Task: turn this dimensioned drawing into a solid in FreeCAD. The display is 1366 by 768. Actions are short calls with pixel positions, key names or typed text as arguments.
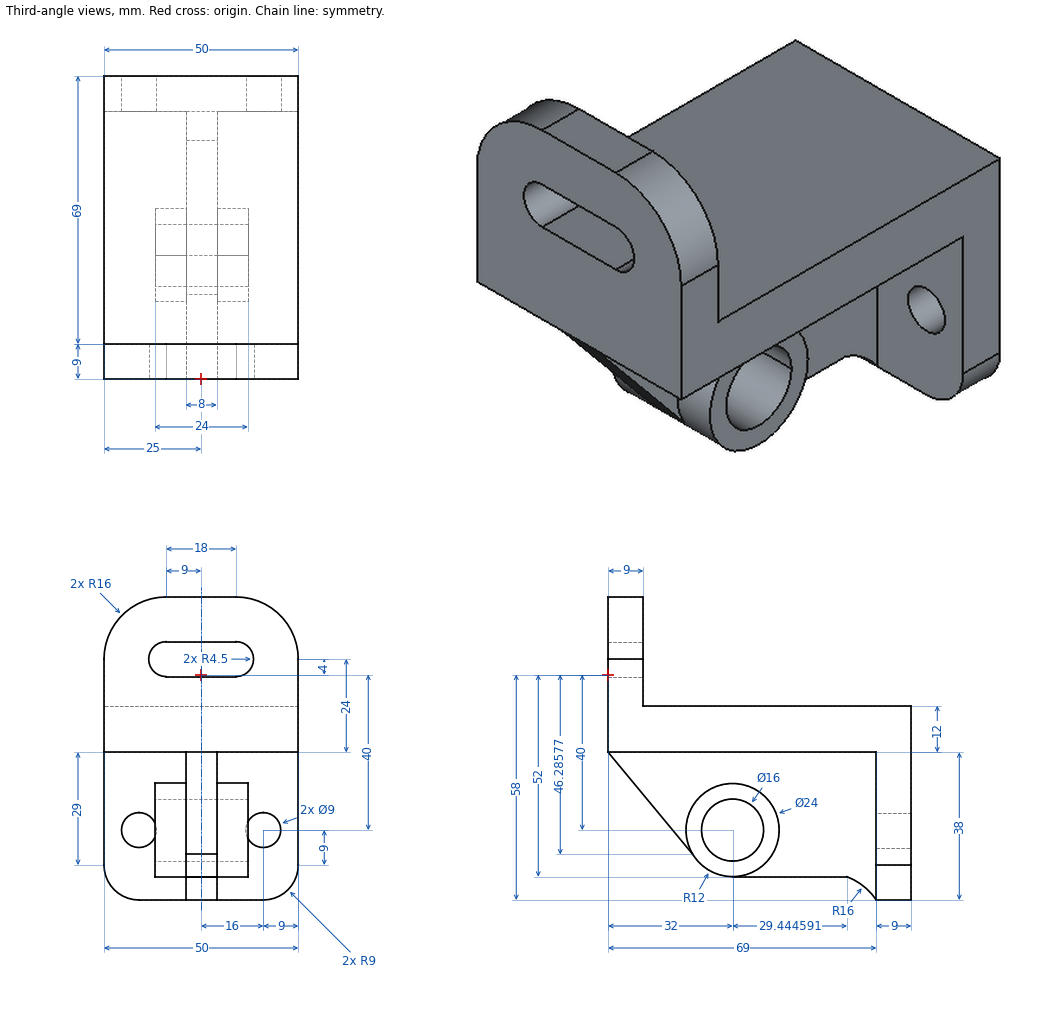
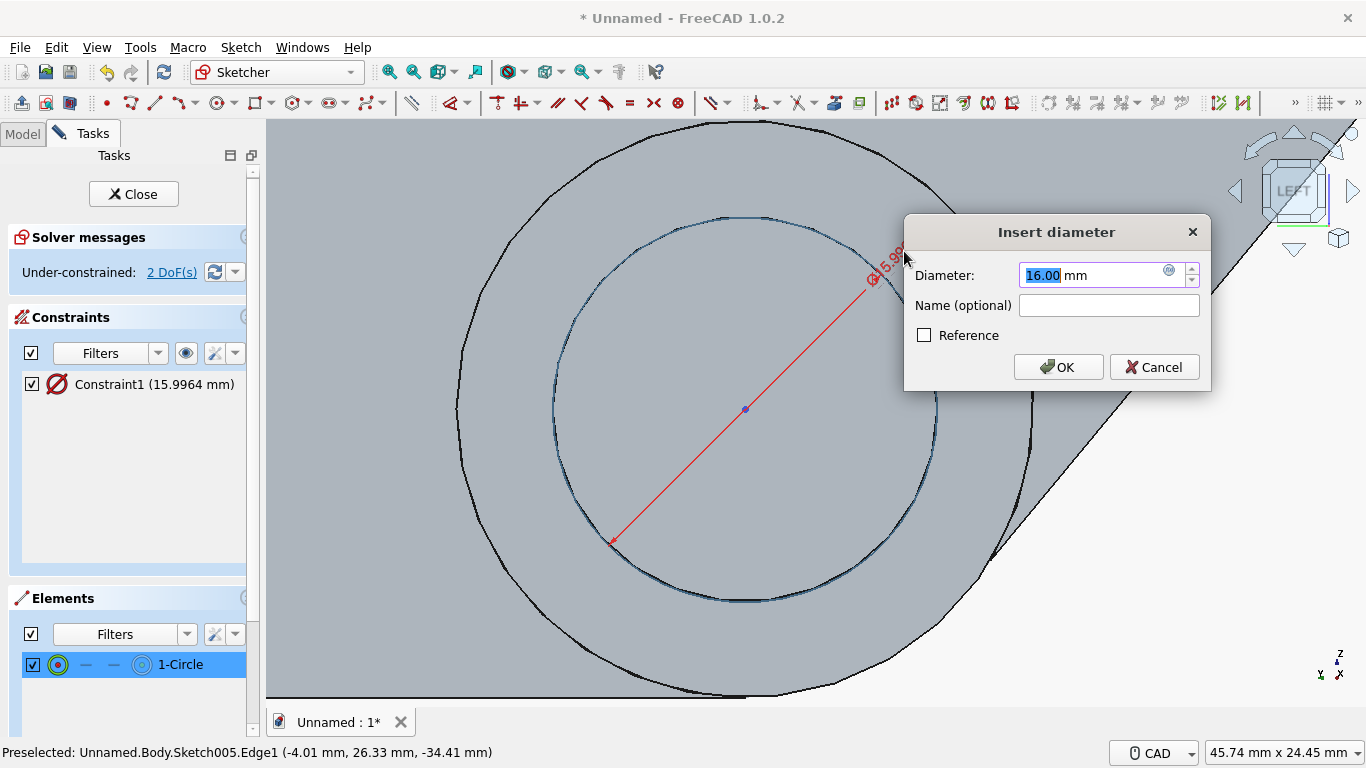
text(16)
key(Return)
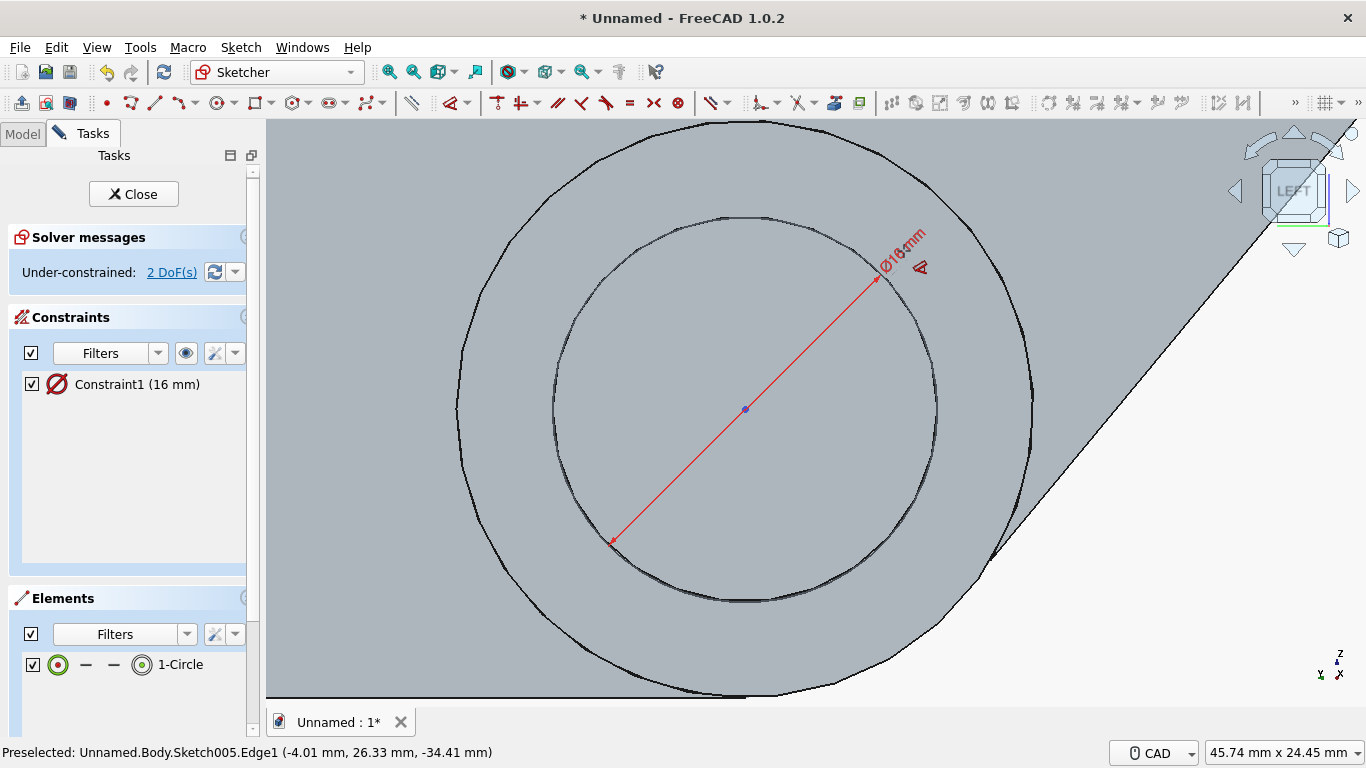
click(745, 410)
click(973, 444)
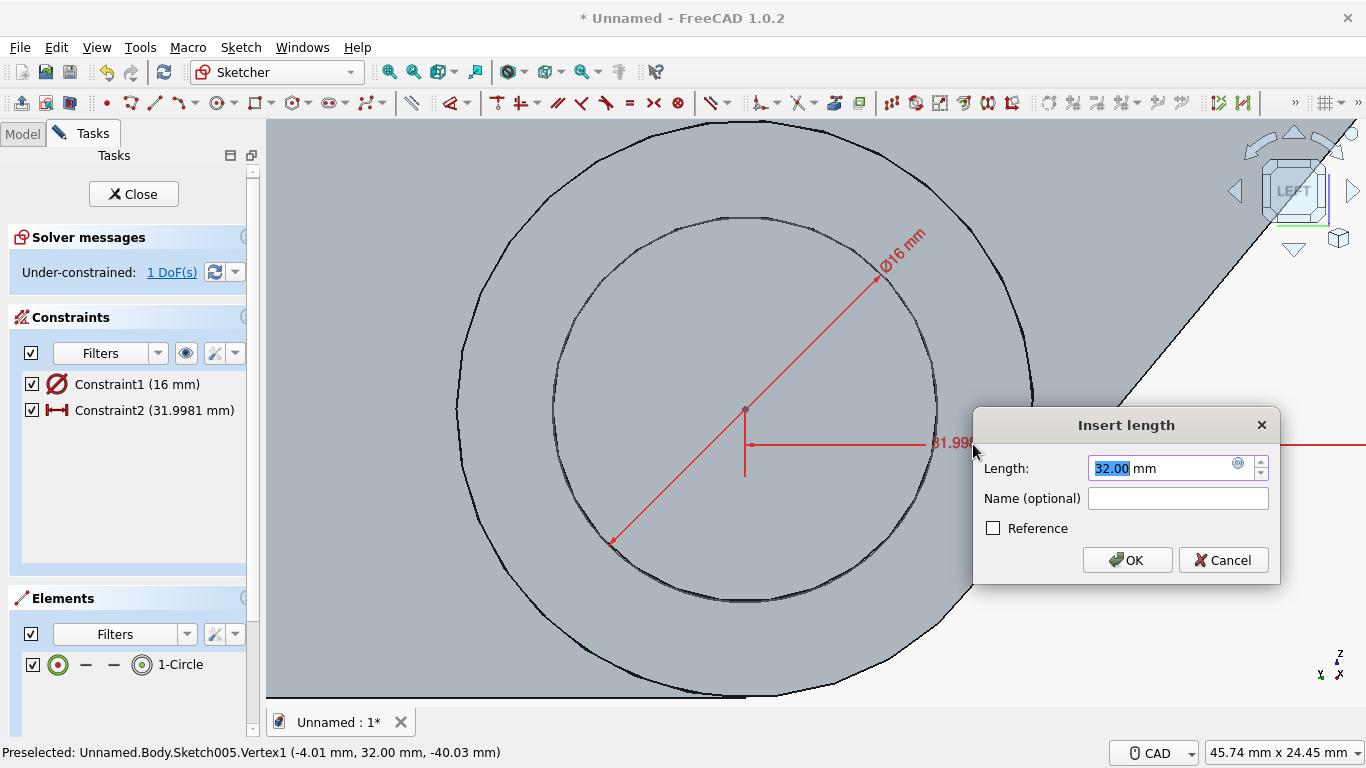
text(32)
key(Return)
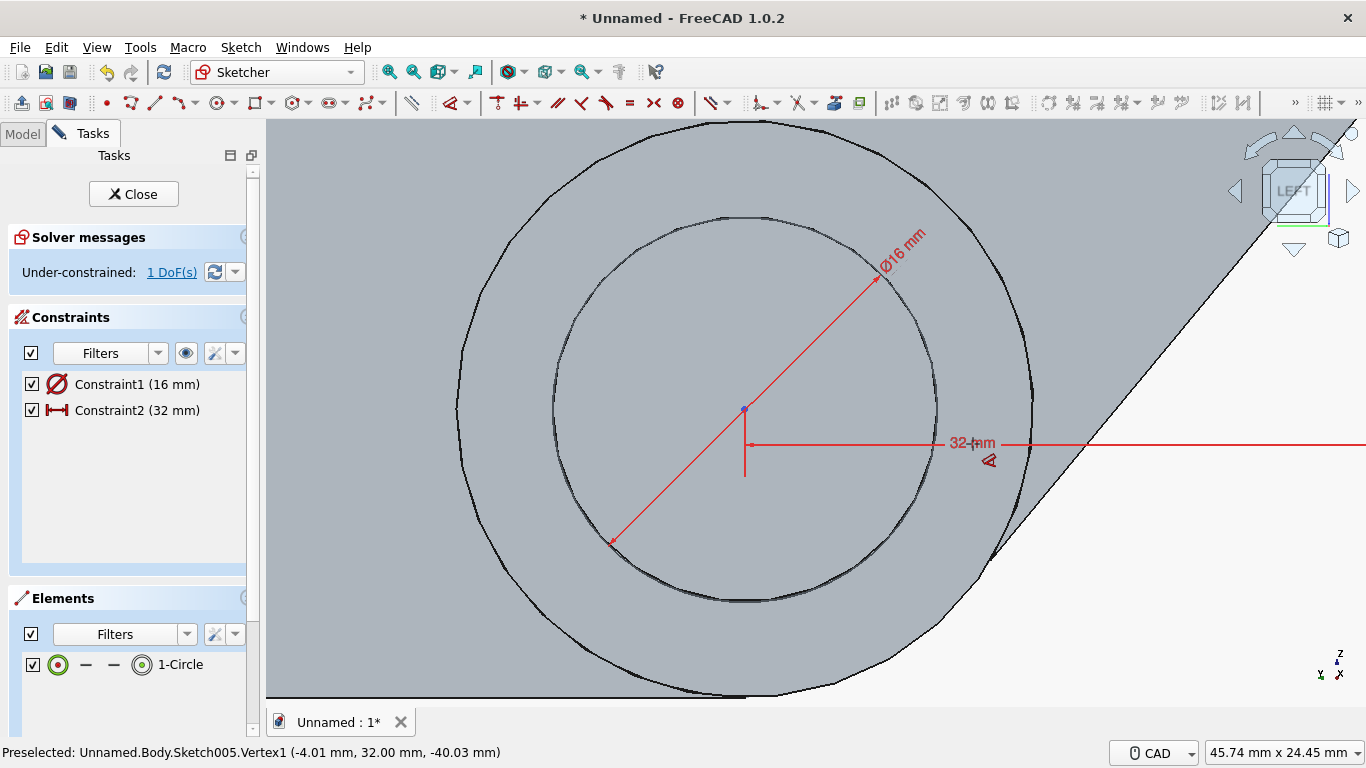
click(745, 410)
click(711, 278)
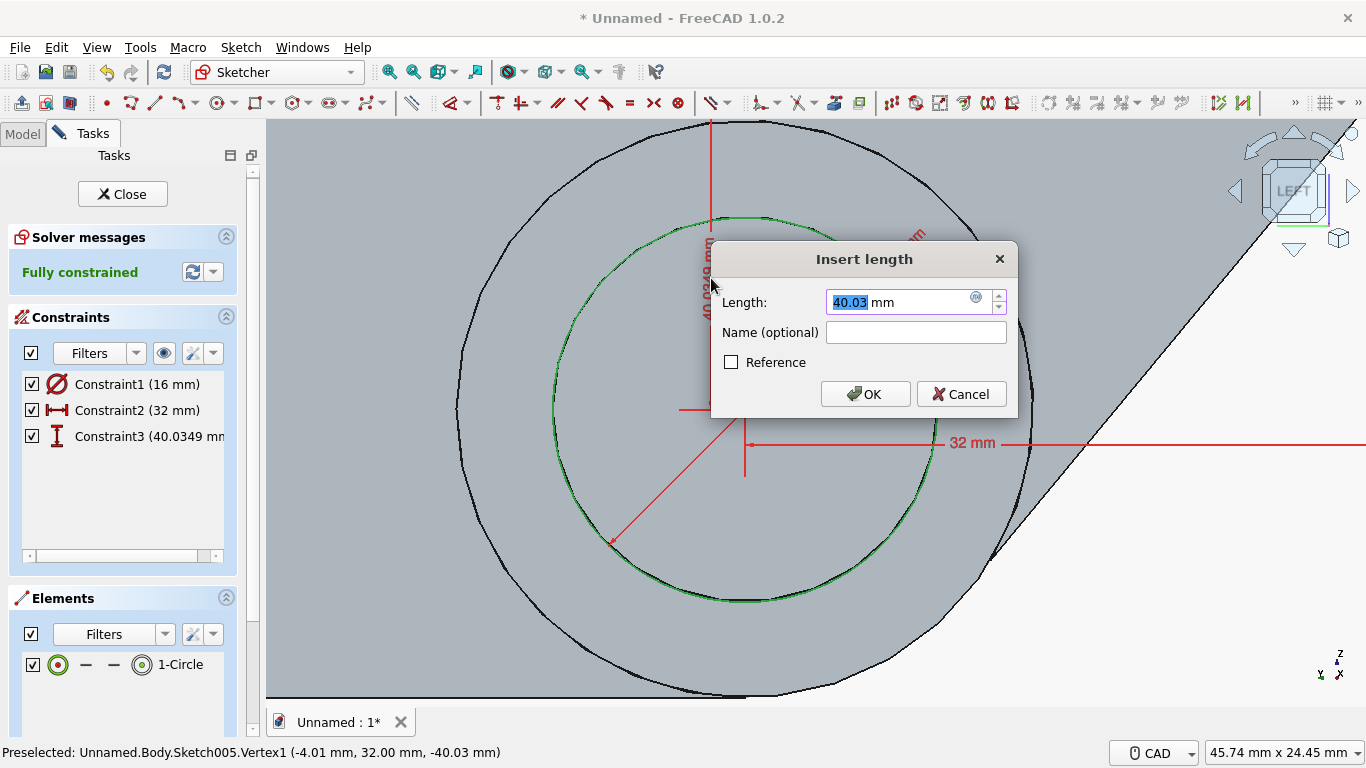
text(40)
key(Return)
key(Escape)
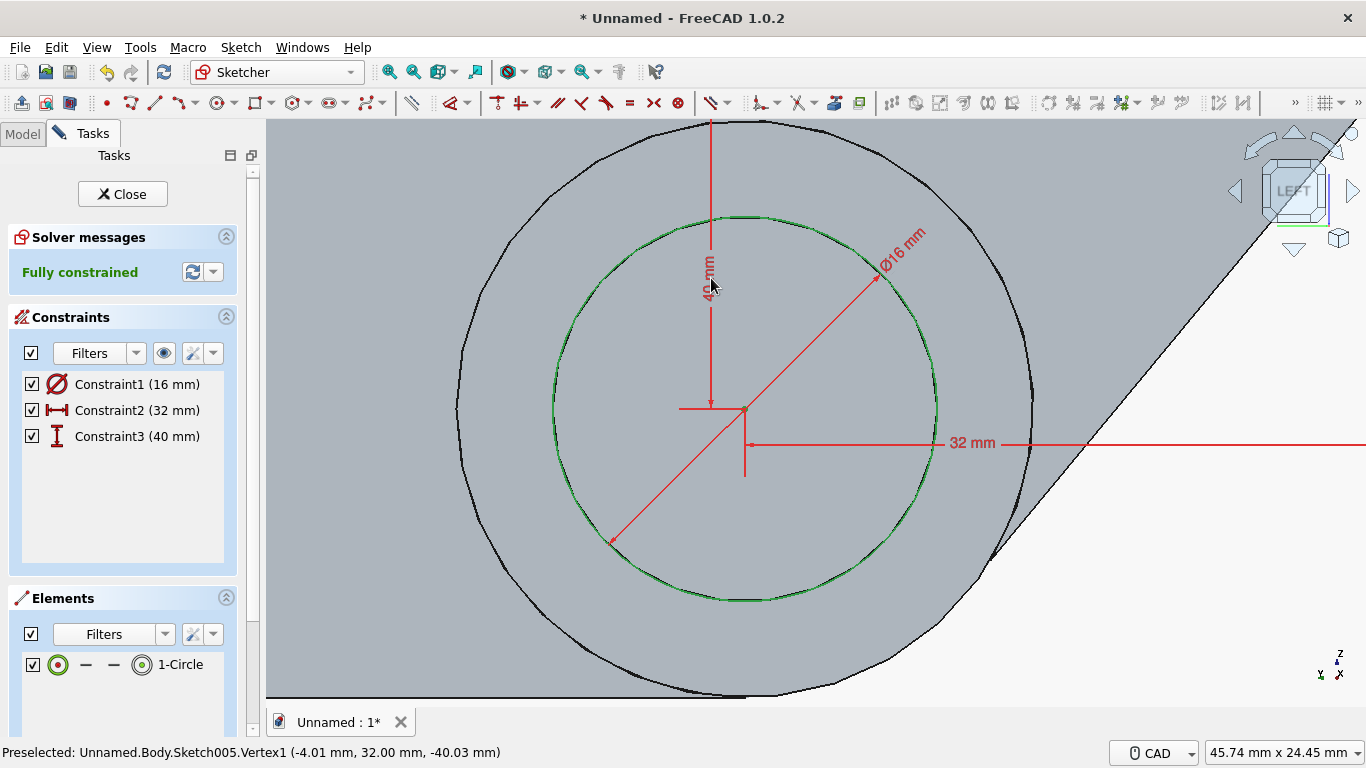
click(123, 194)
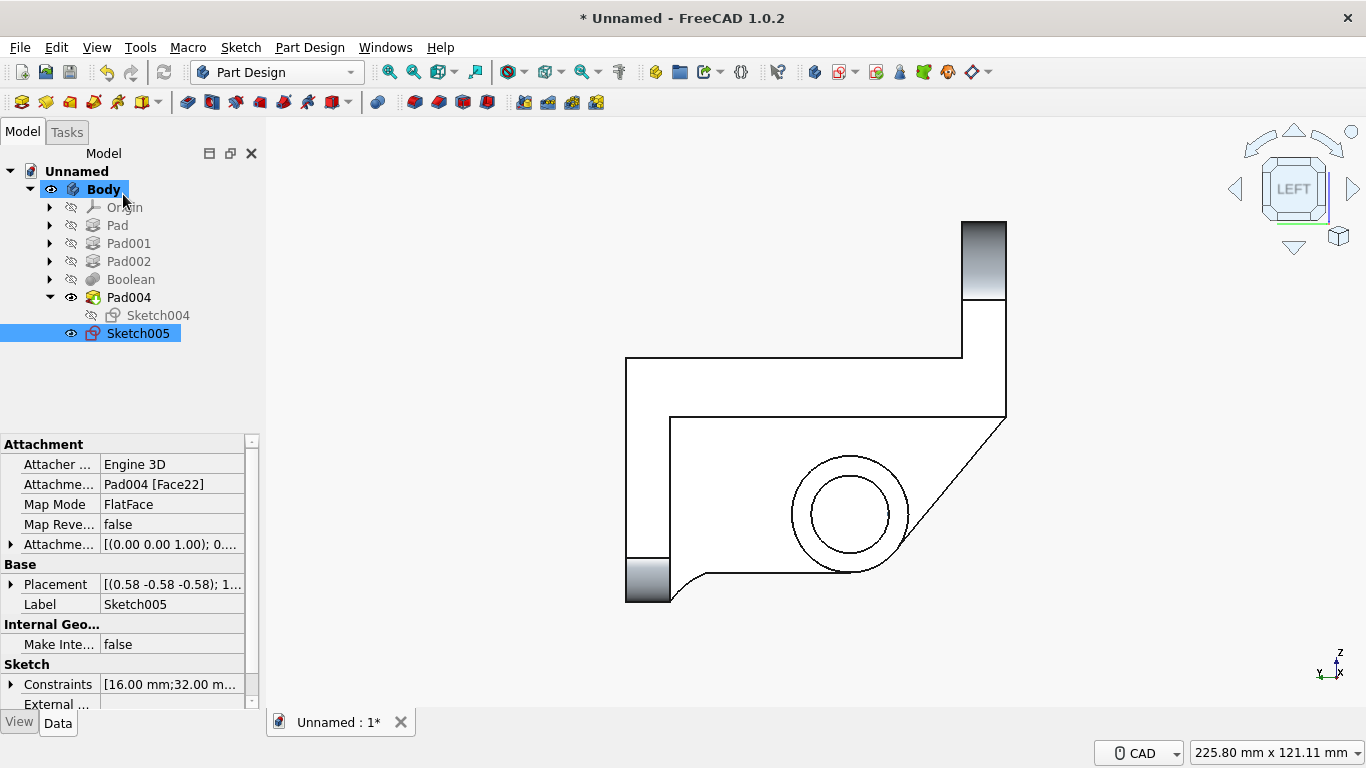
click(188, 102)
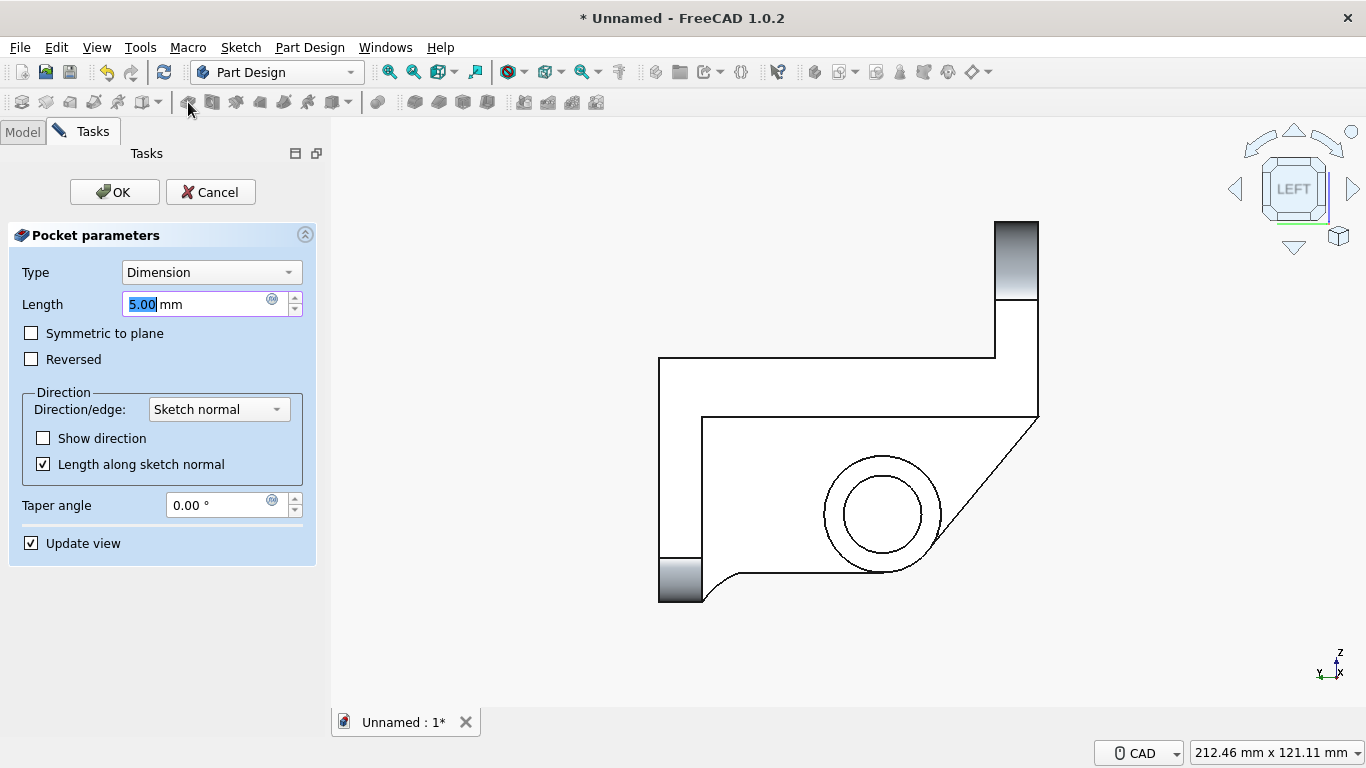
click(212, 272)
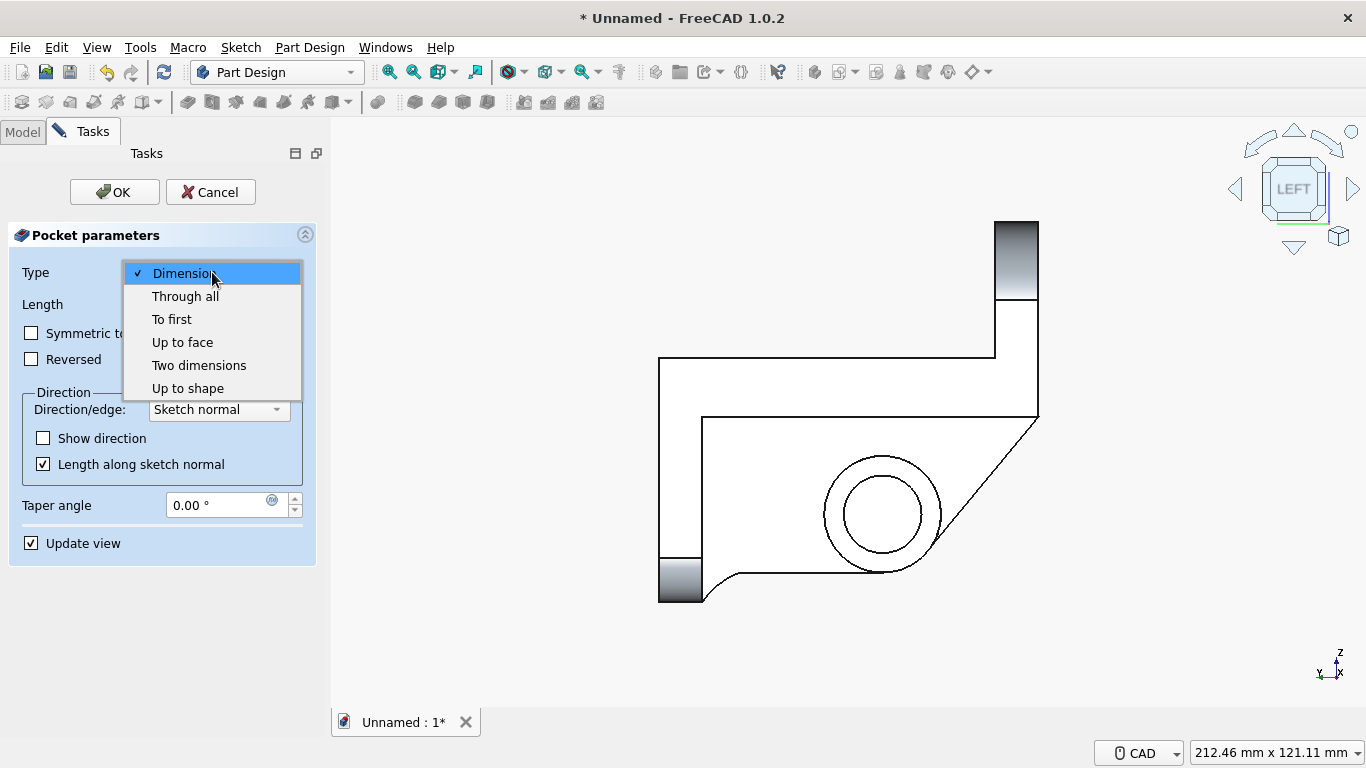
click(212, 296)